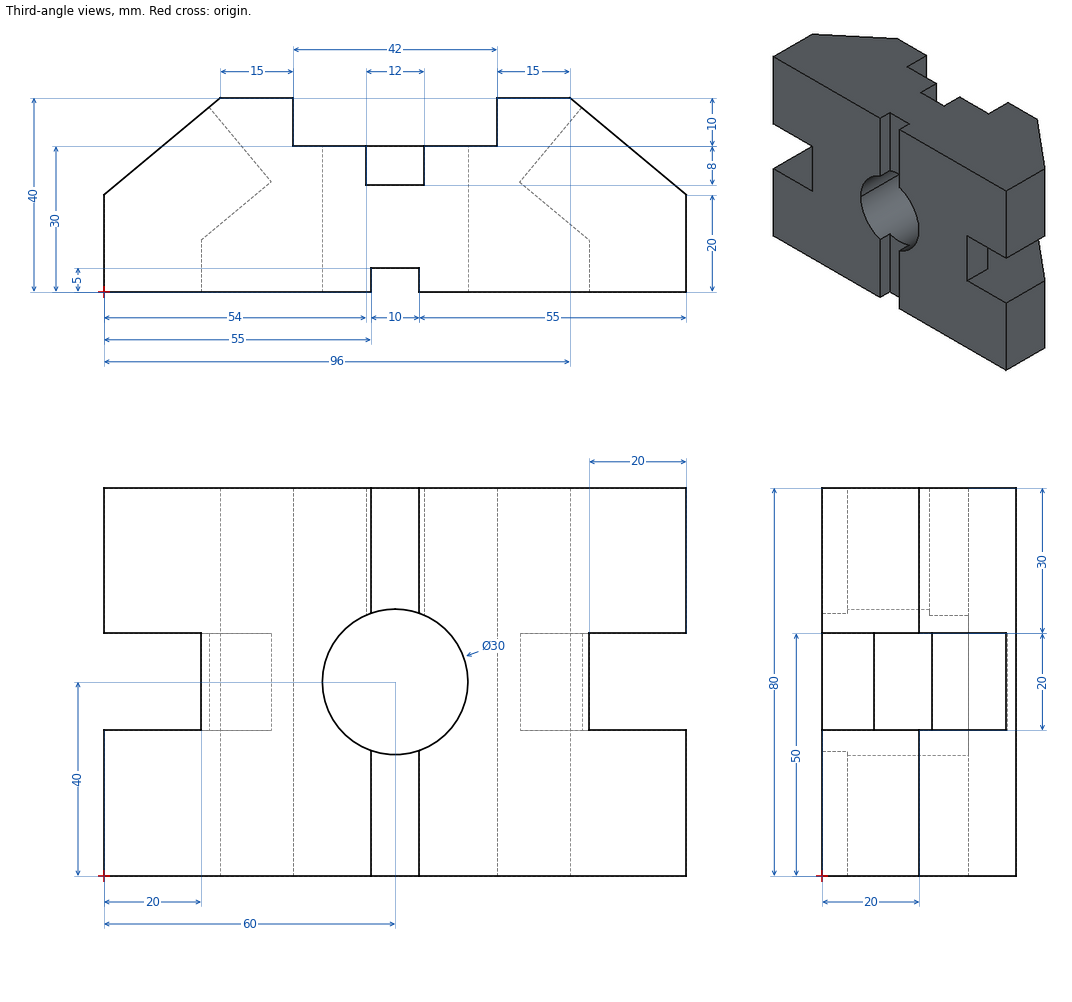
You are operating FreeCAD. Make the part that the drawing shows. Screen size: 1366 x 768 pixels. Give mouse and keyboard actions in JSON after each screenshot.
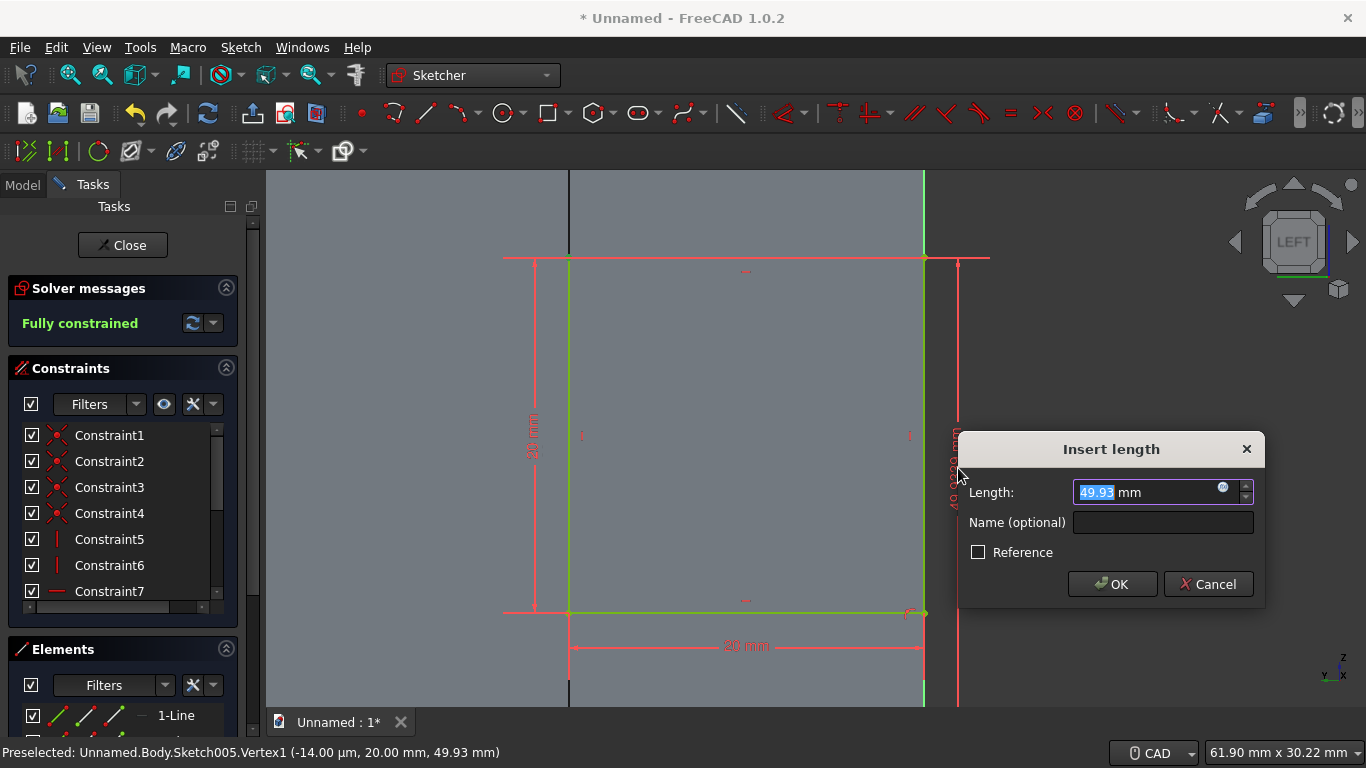
{"action": "type", "text": "50"}
{"action": "key", "text": "Return"}
{"action": "key", "text": "Escape"}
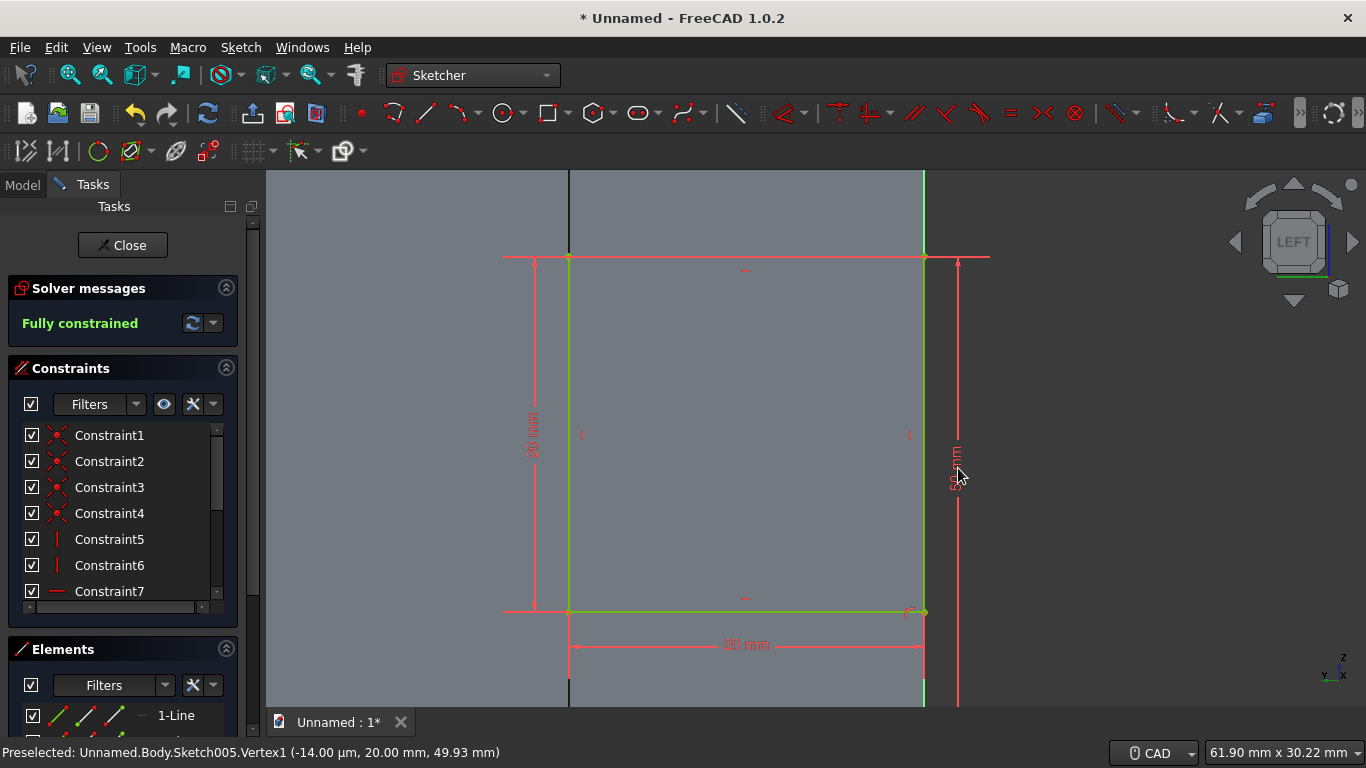
{"action": "left_click", "coordinate": [123, 245]}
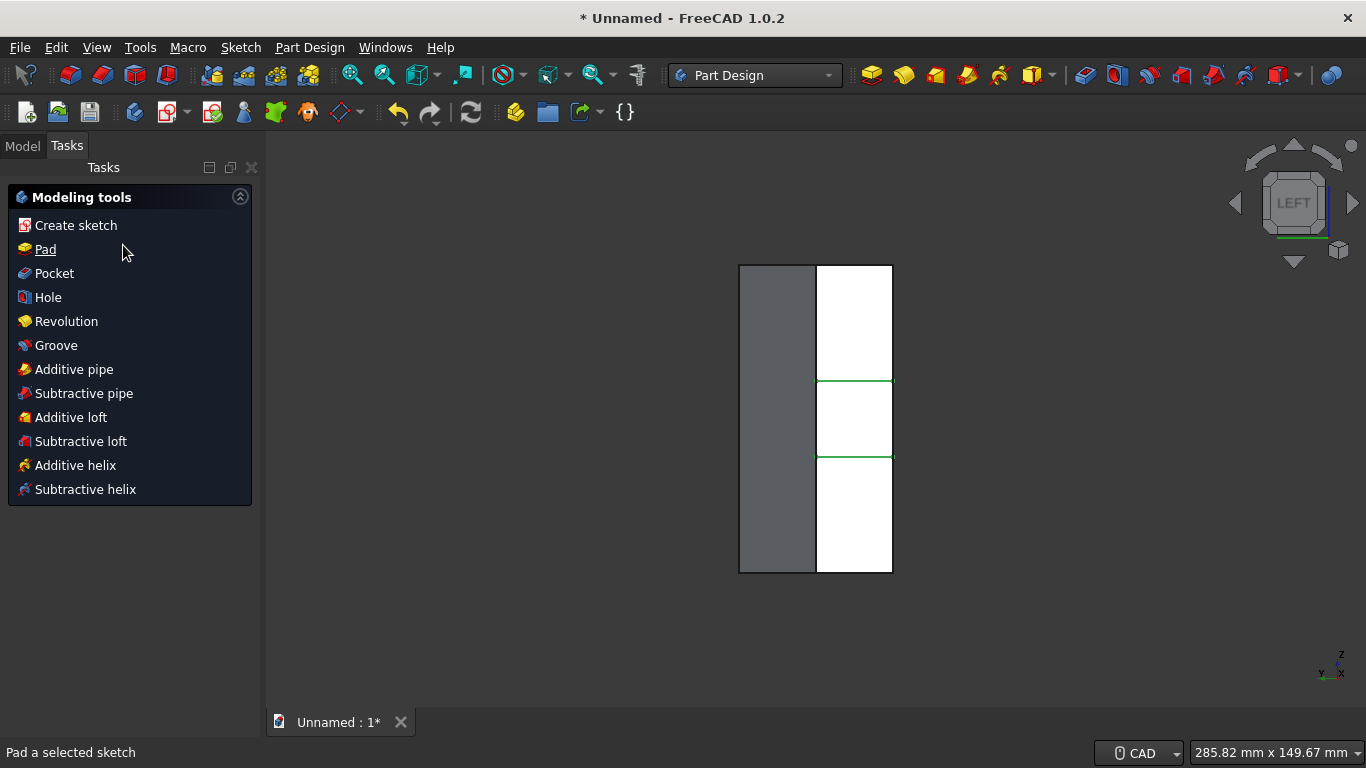
{"action": "left_click", "coordinate": [1086, 76]}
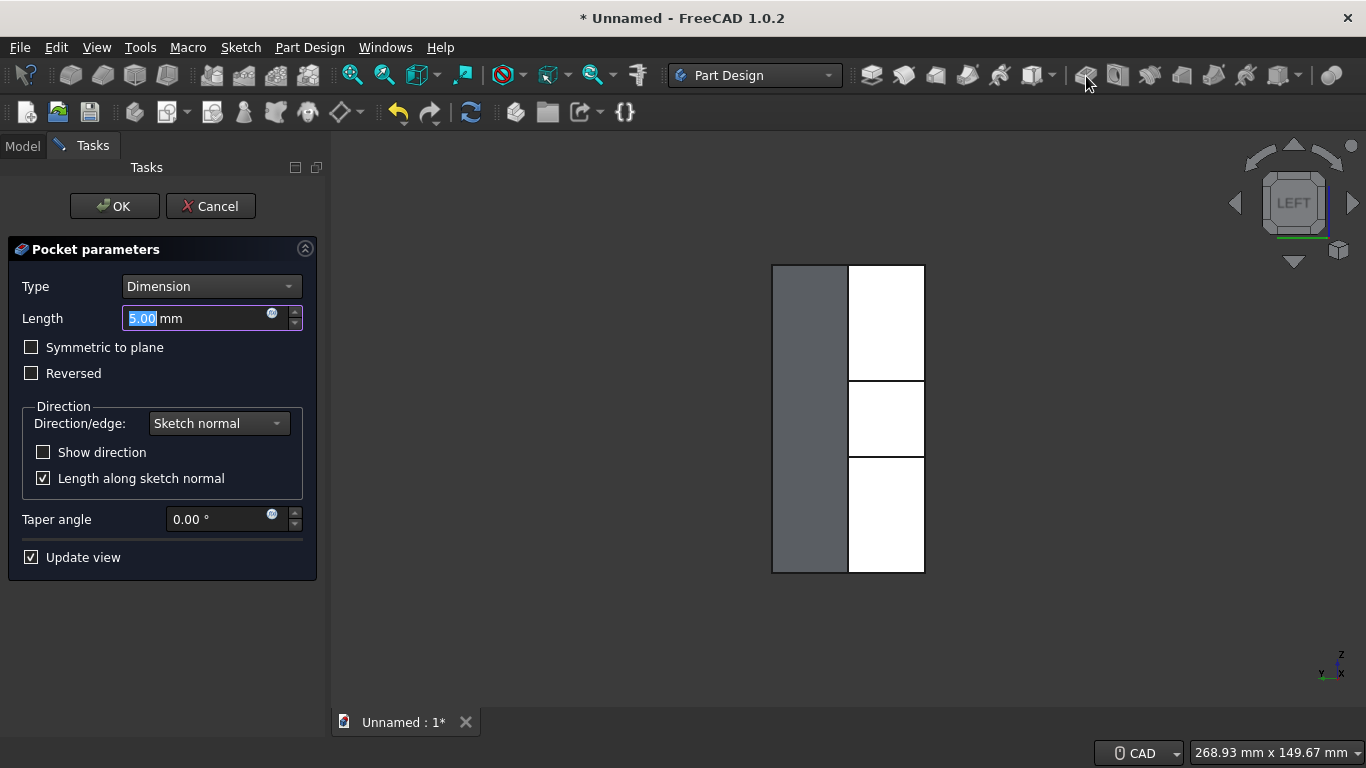
{"action": "type", "text": "20"}
{"action": "key", "text": "Tab"}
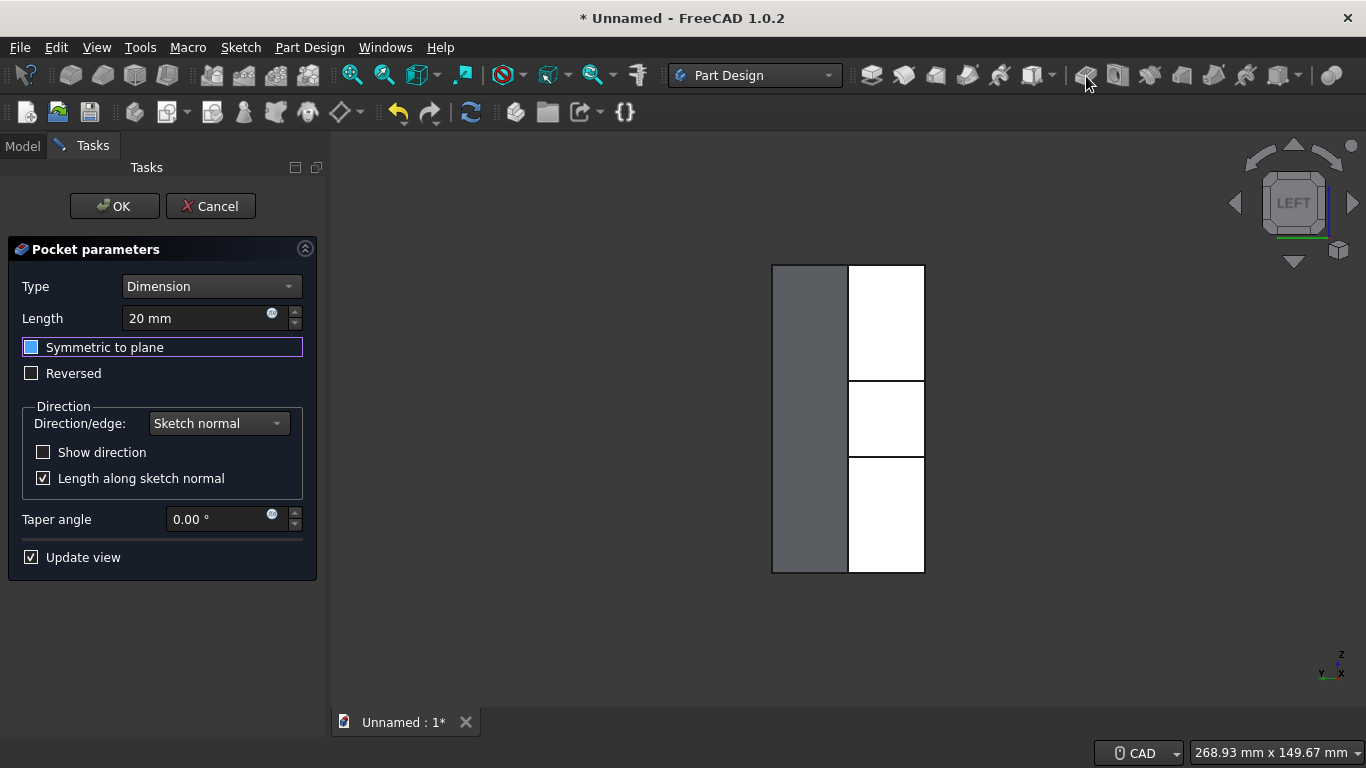
{"action": "left_click", "coordinate": [115, 206]}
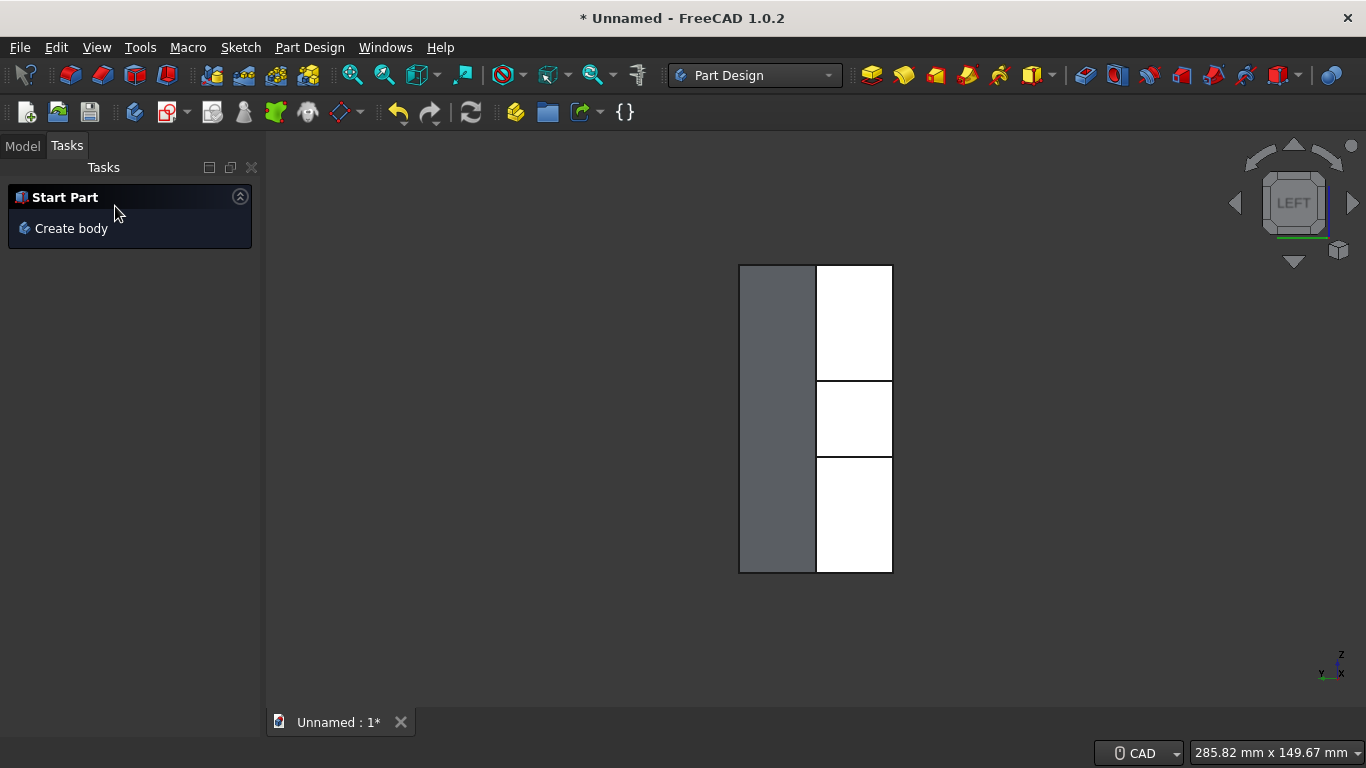
{"action": "left_click", "coordinate": [778, 330]}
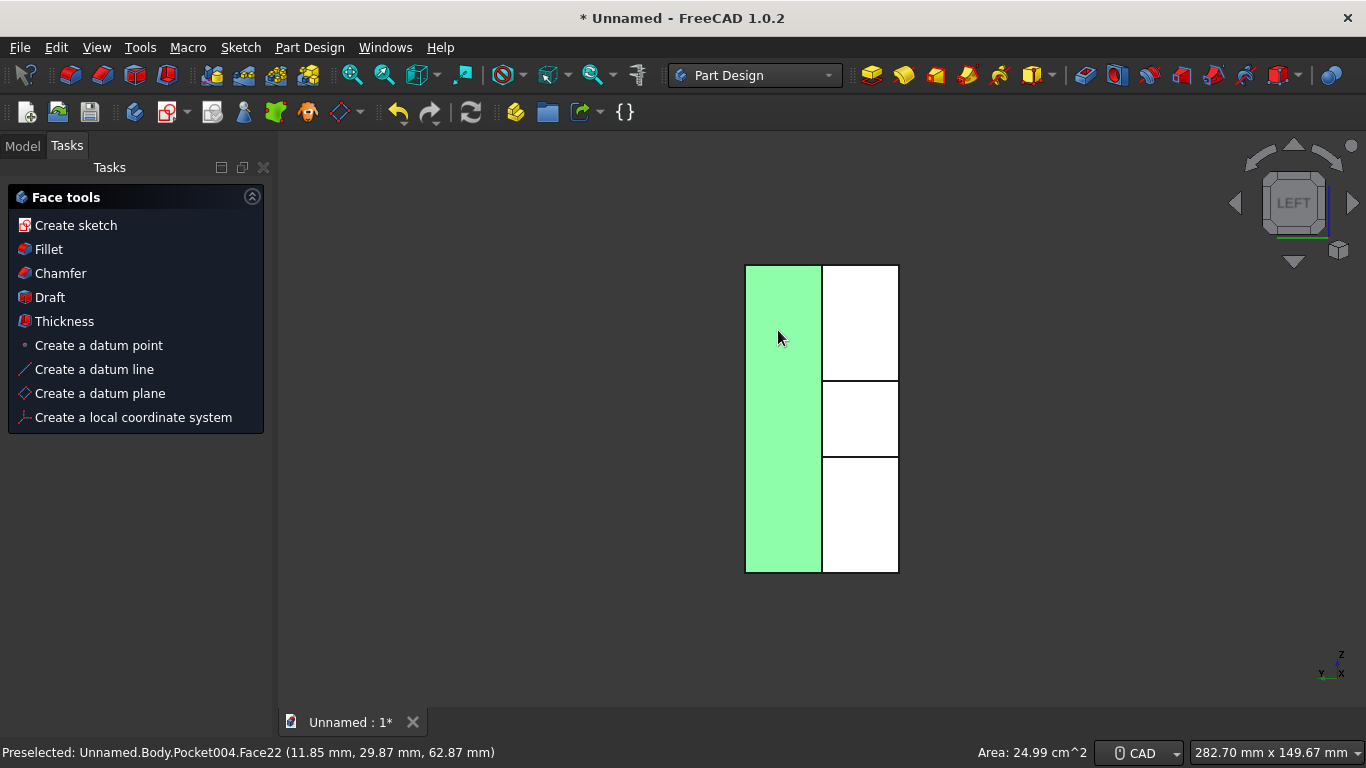
{"action": "left_click", "coordinate": [168, 112]}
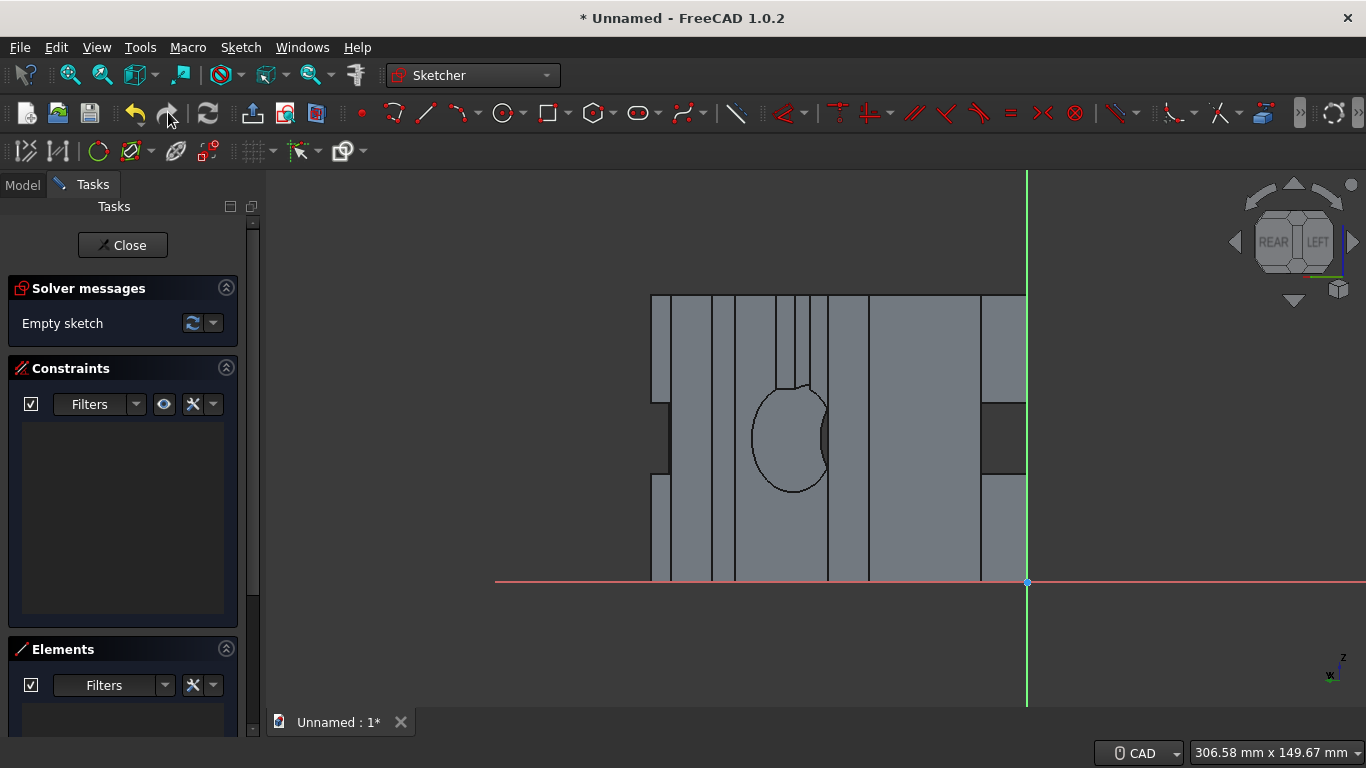
{"action": "scroll", "coordinate": [1201, 558], "scroll_direction": "up", "scroll_amount": 3}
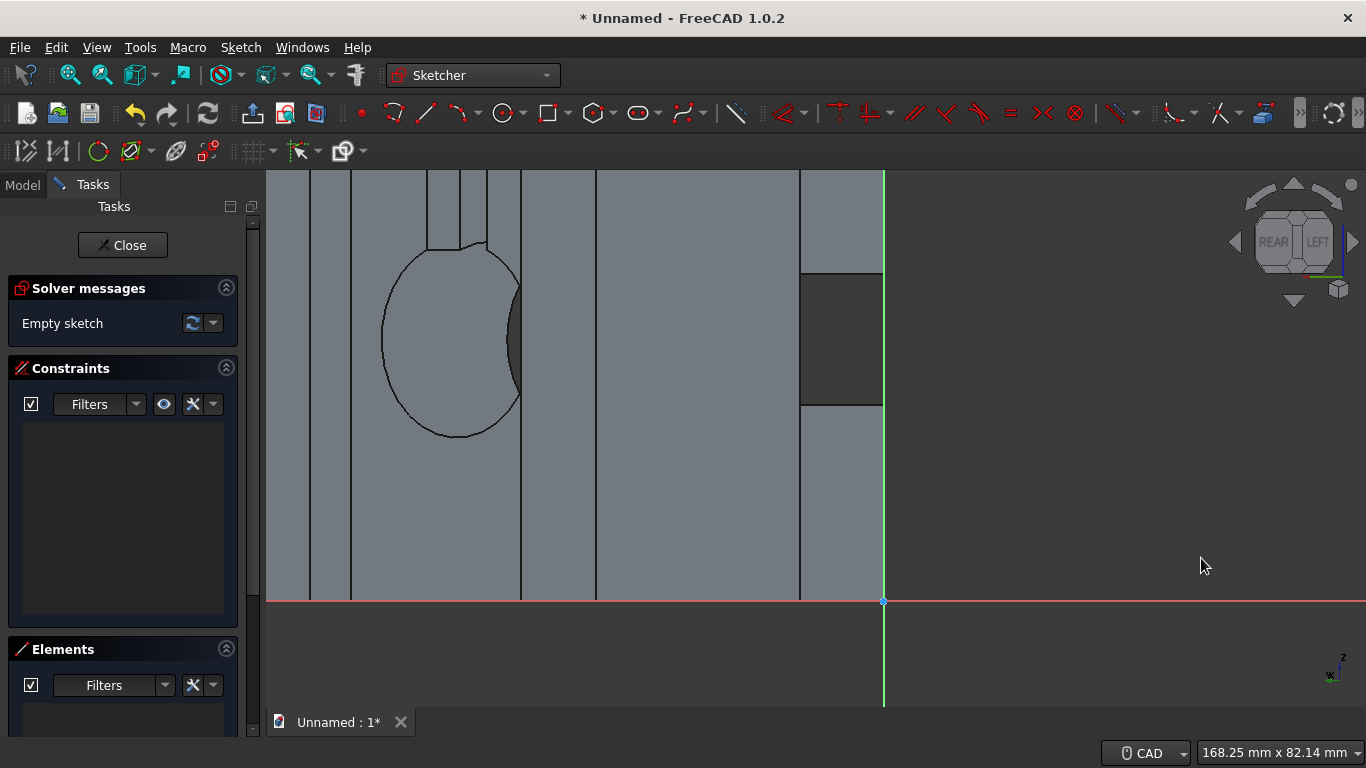
{"action": "key", "text": "g r"}